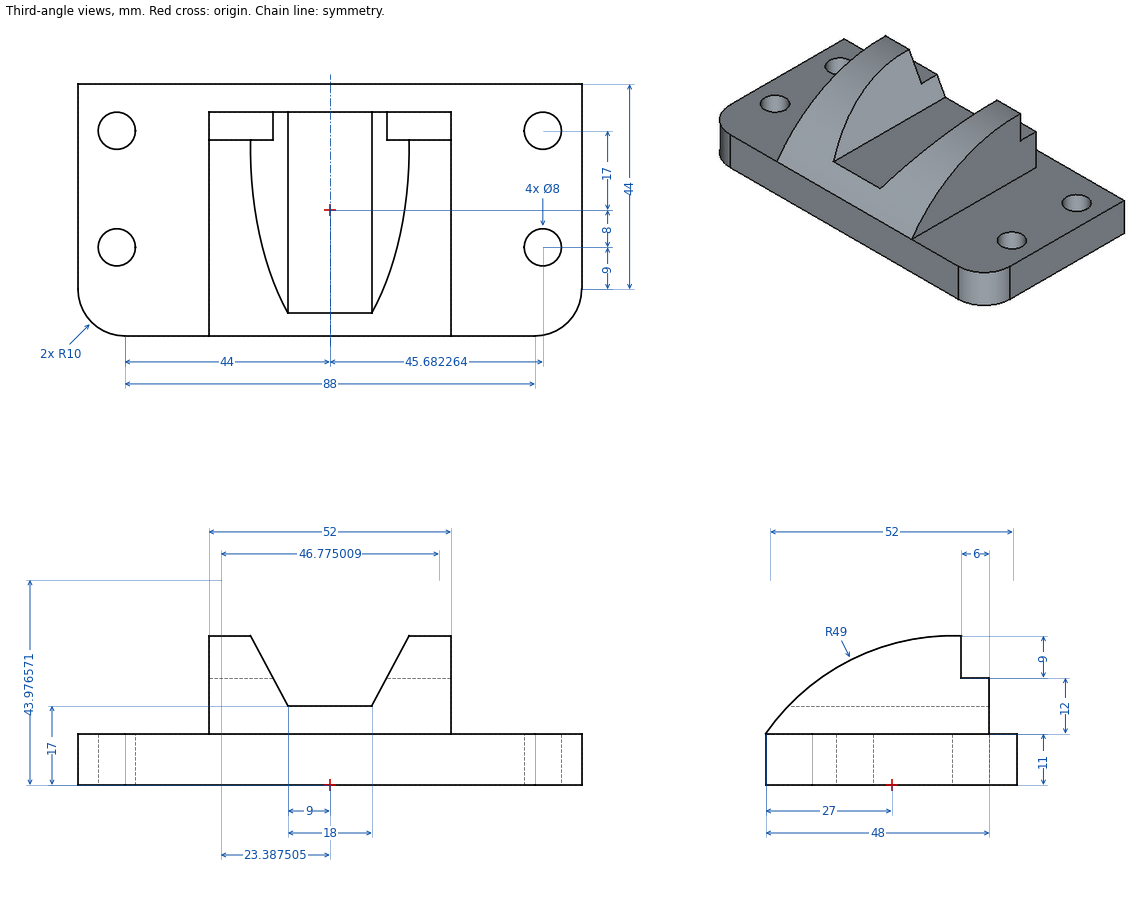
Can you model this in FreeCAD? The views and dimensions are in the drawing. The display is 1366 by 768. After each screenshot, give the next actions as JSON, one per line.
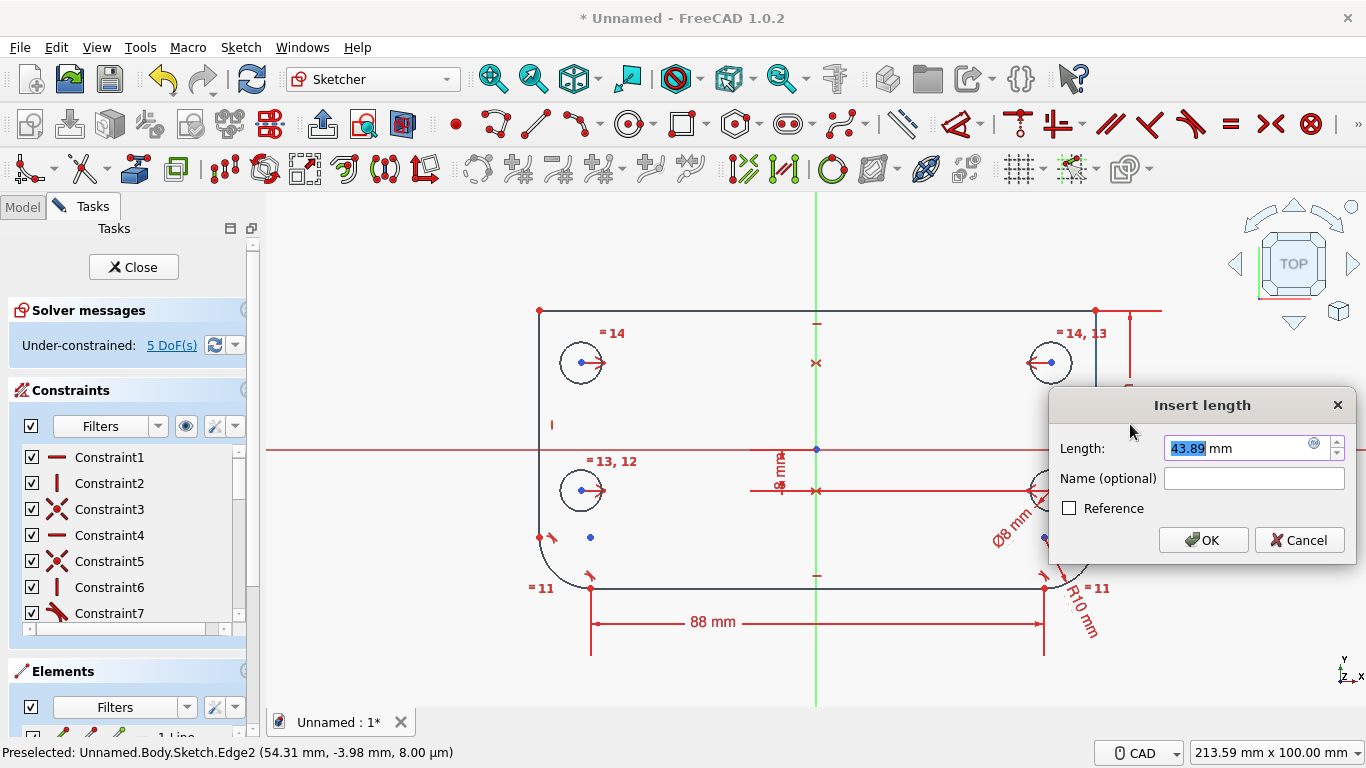
{"action": "type", "text": "44"}
{"action": "key", "text": "Return"}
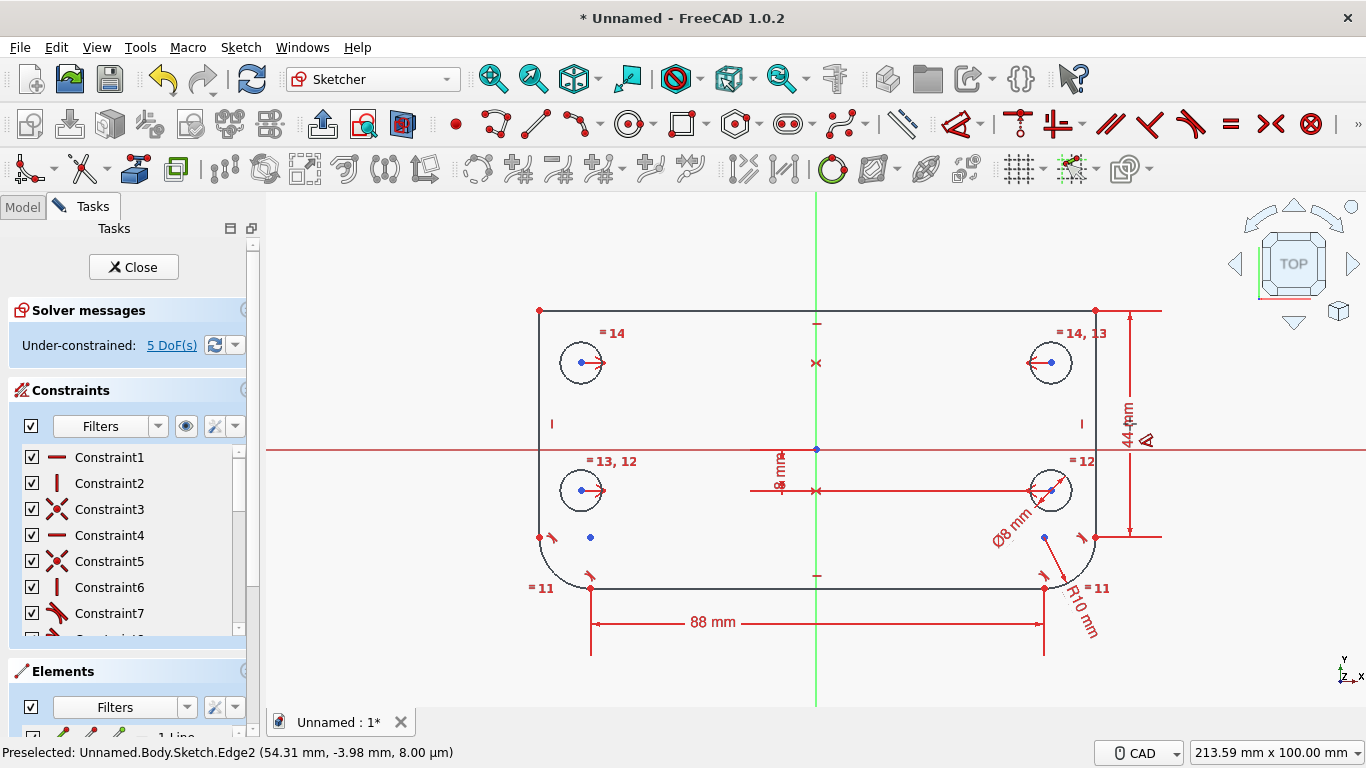
{"action": "left_click", "coordinate": [1051, 363]}
{"action": "left_click", "coordinate": [782, 406]}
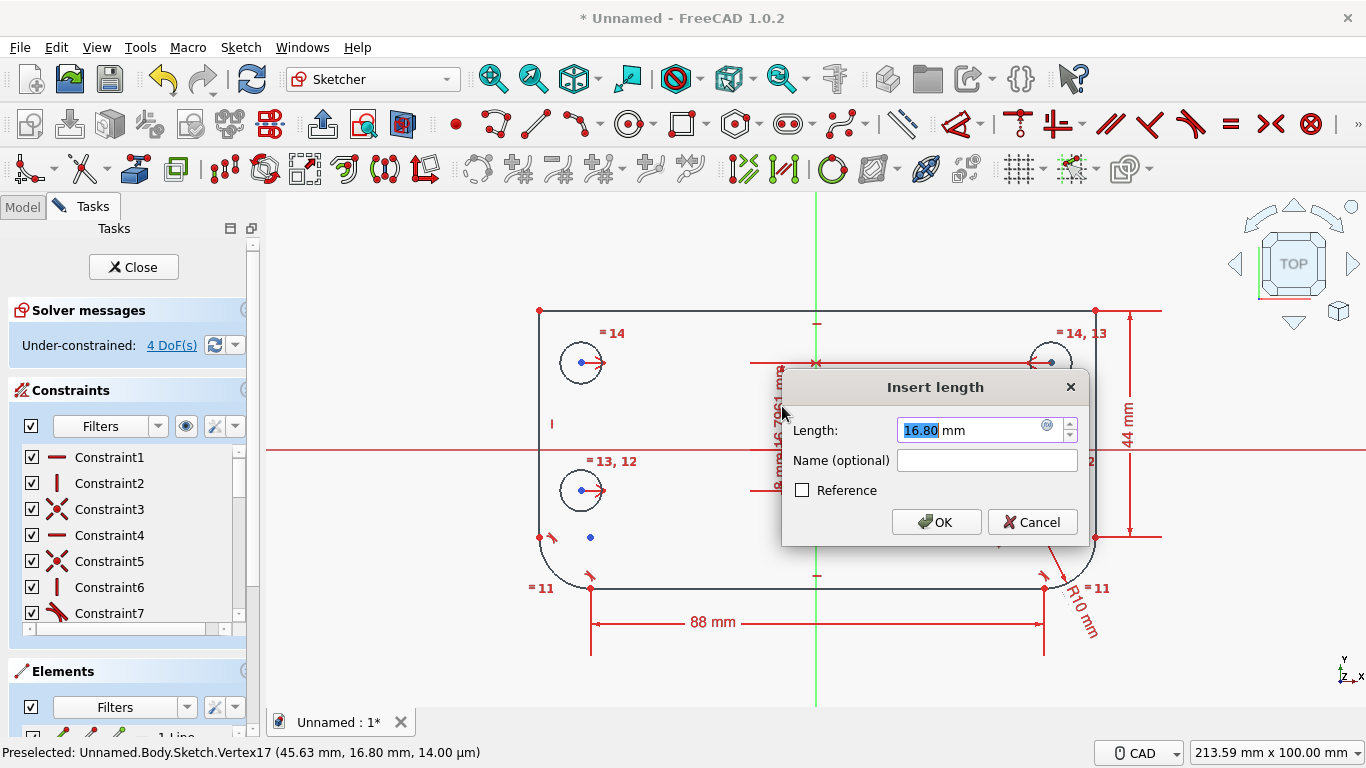
{"action": "type", "text": "17"}
{"action": "key", "text": "Return"}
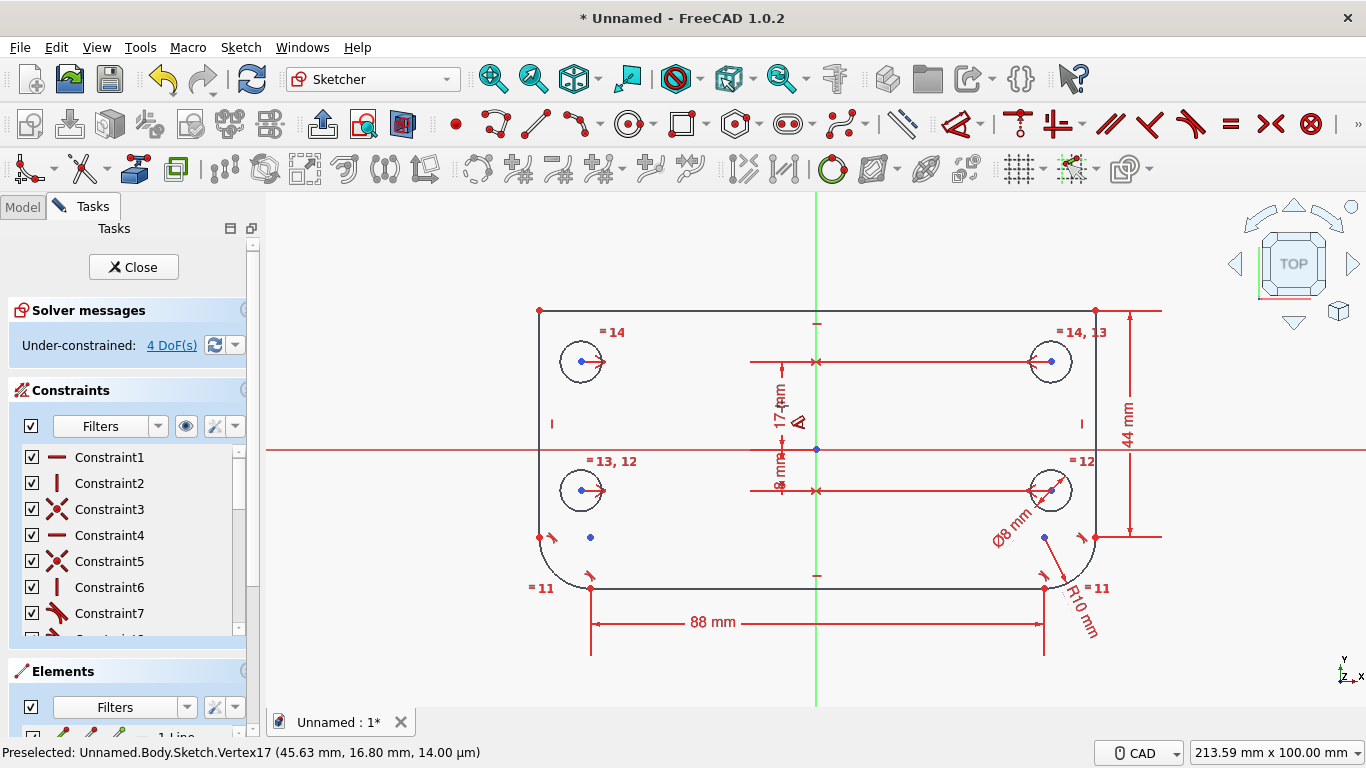
{"action": "left_click", "coordinate": [1096, 537]}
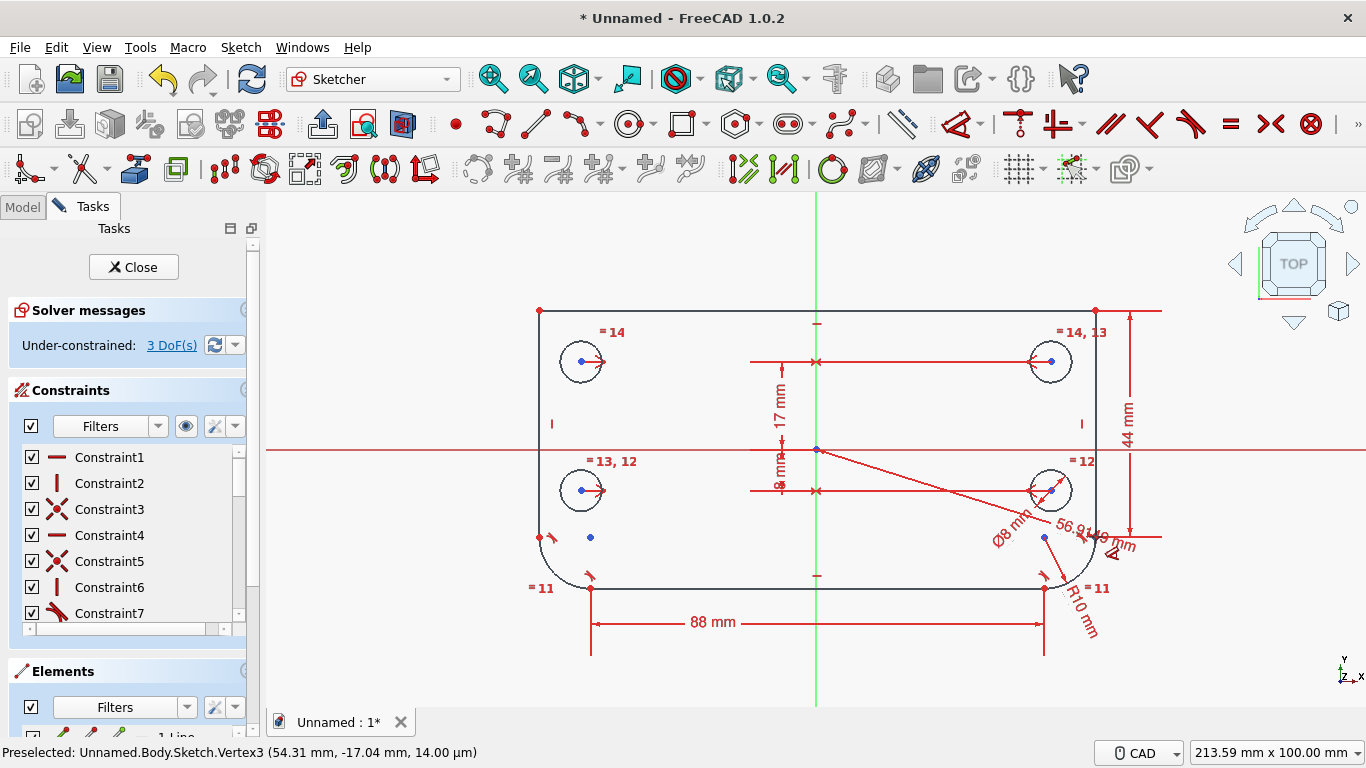
{"action": "left_click", "coordinate": [1051, 491]}
{"action": "left_click", "coordinate": [1130, 514]}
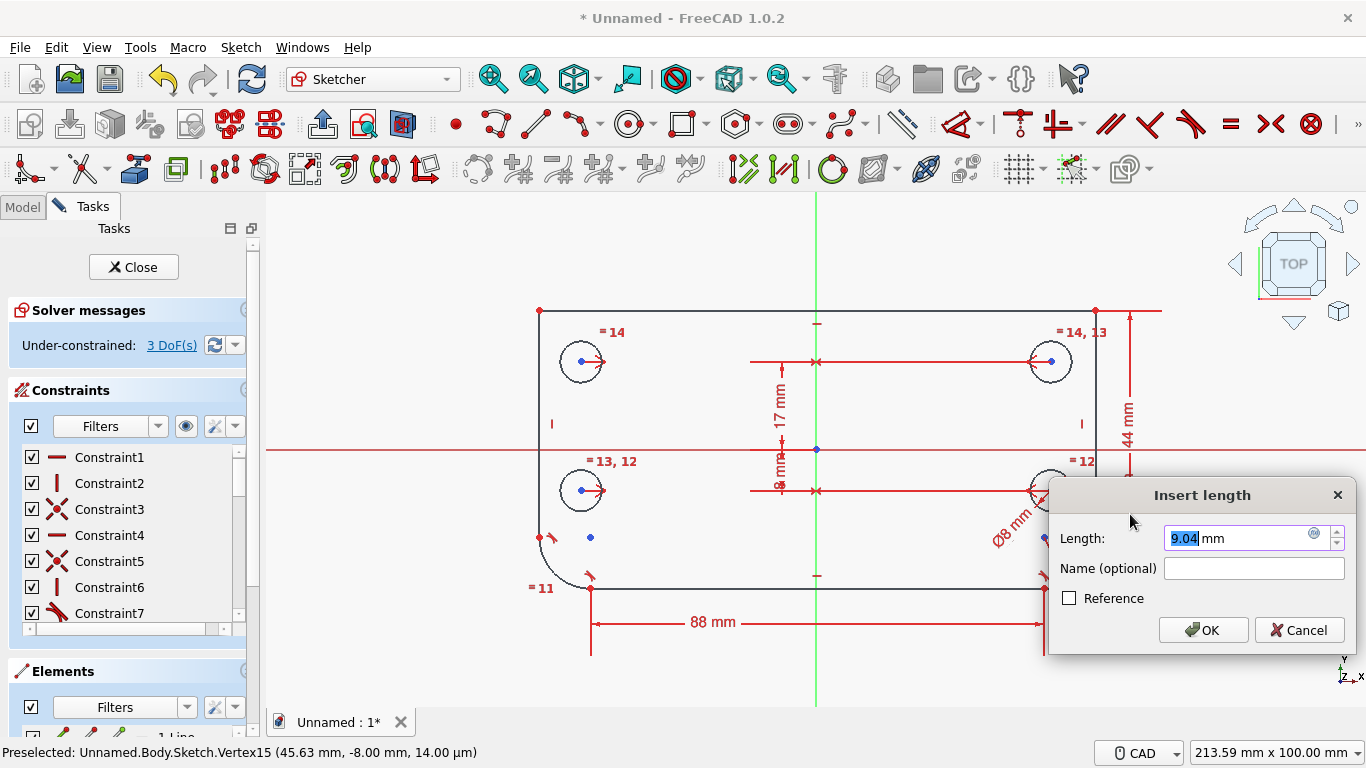
{"action": "type", "text": "9"}
{"action": "key", "text": "Return"}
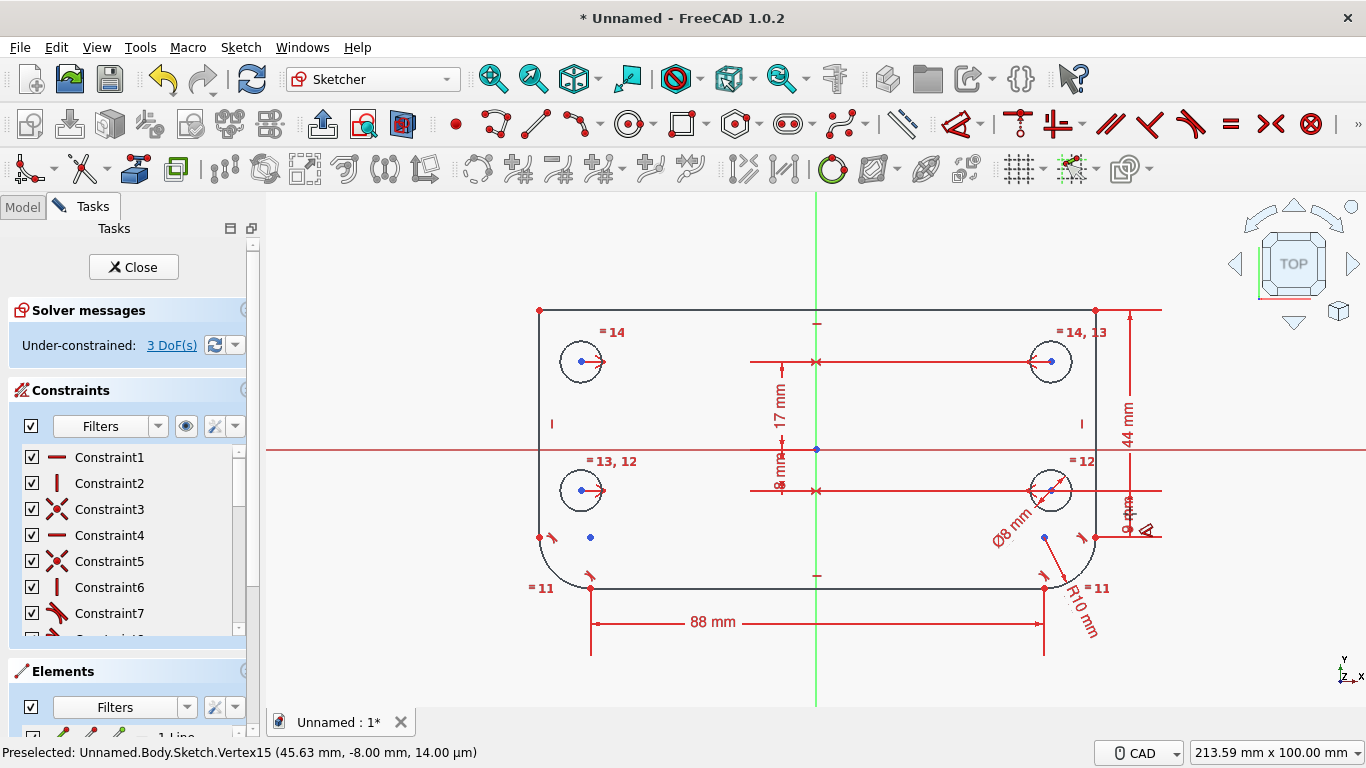
{"action": "left_click", "coordinate": [591, 589]}
{"action": "left_click", "coordinate": [625, 623]}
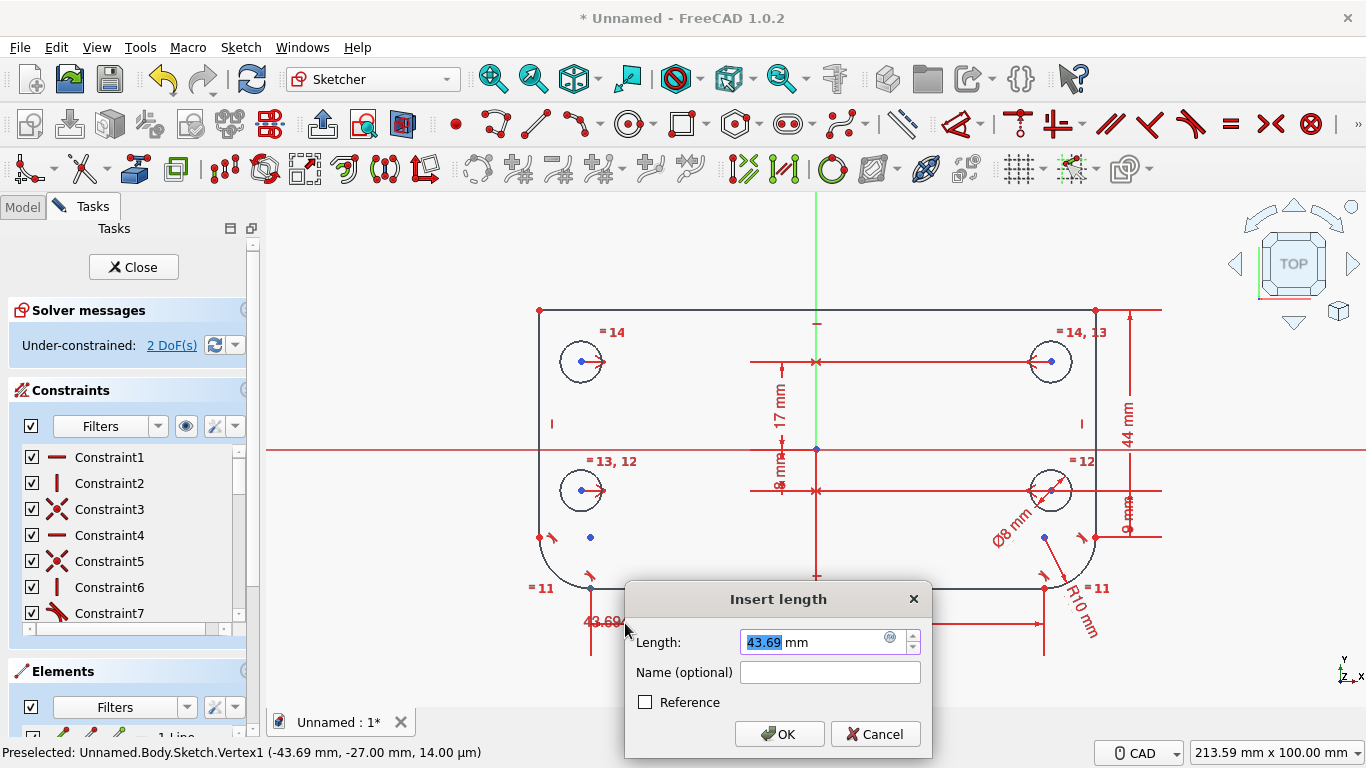
{"action": "type", "text": "44"}
{"action": "key", "text": "Return"}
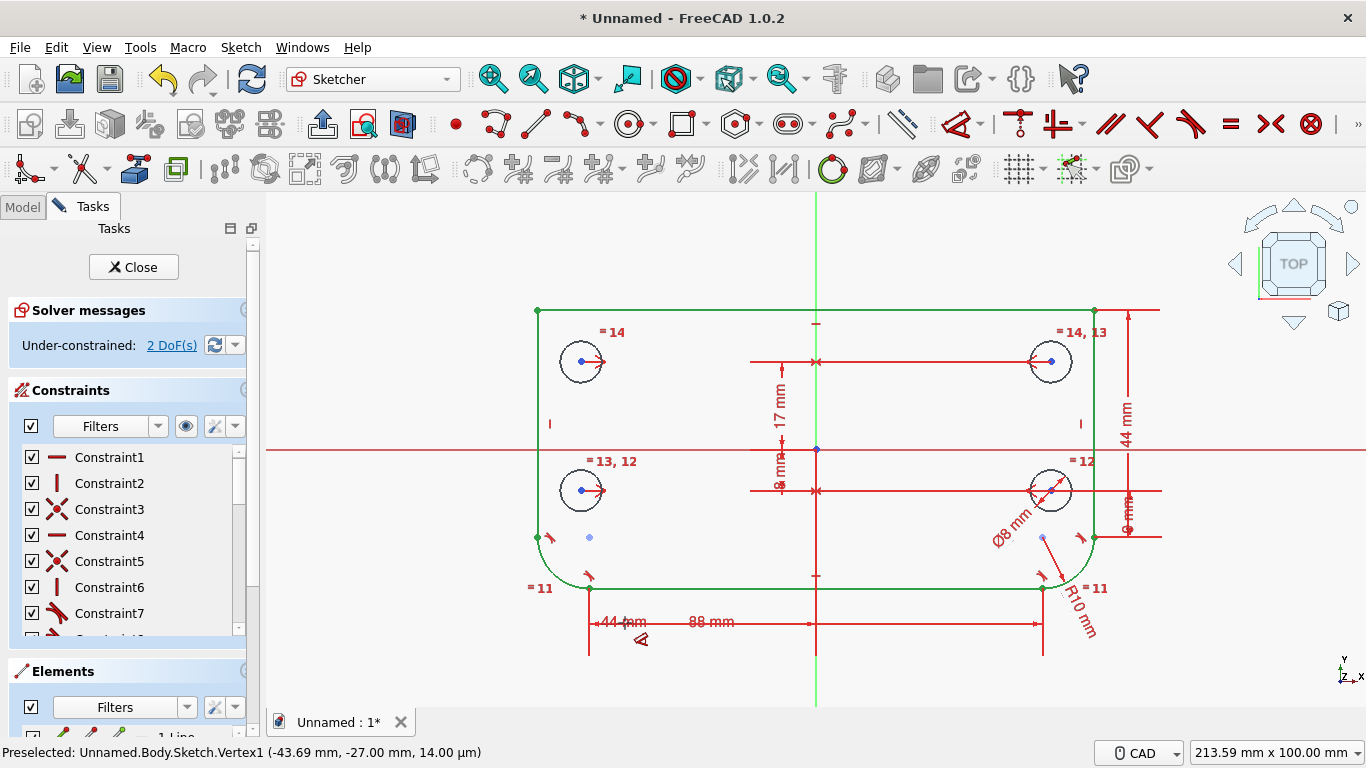
{"action": "left_click", "coordinate": [1051, 491]}
{"action": "left_click", "coordinate": [934, 525]}